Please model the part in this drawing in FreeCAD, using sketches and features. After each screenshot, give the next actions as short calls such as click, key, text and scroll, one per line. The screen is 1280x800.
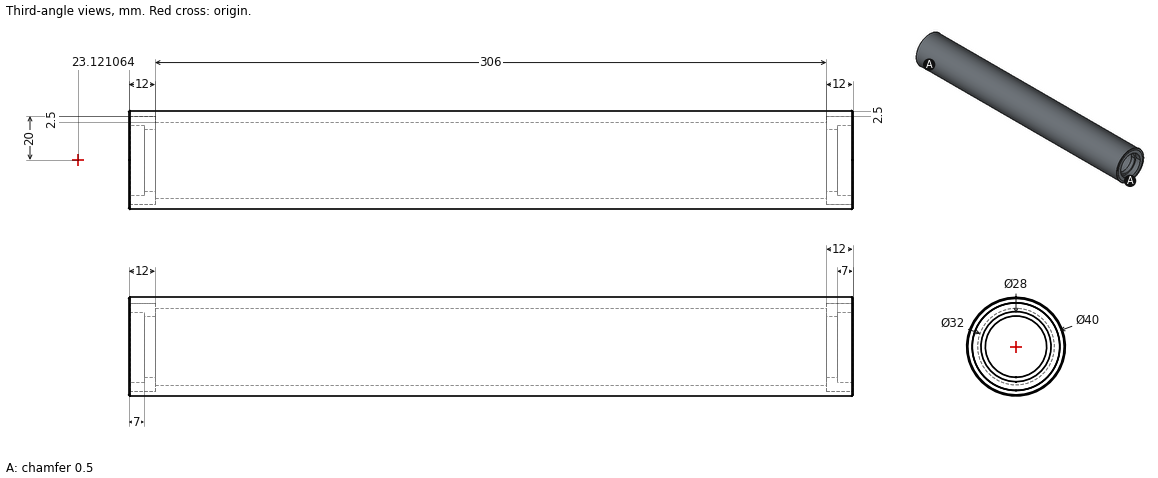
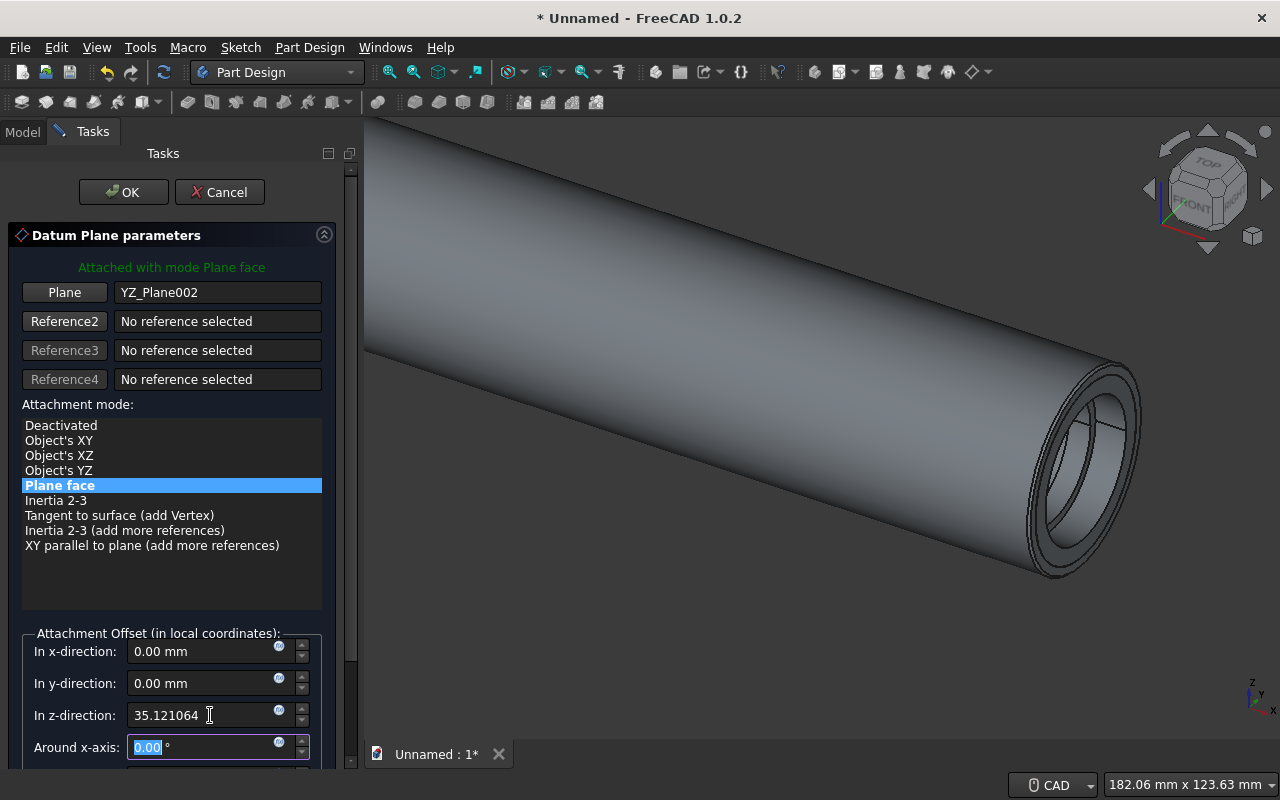
click(124, 192)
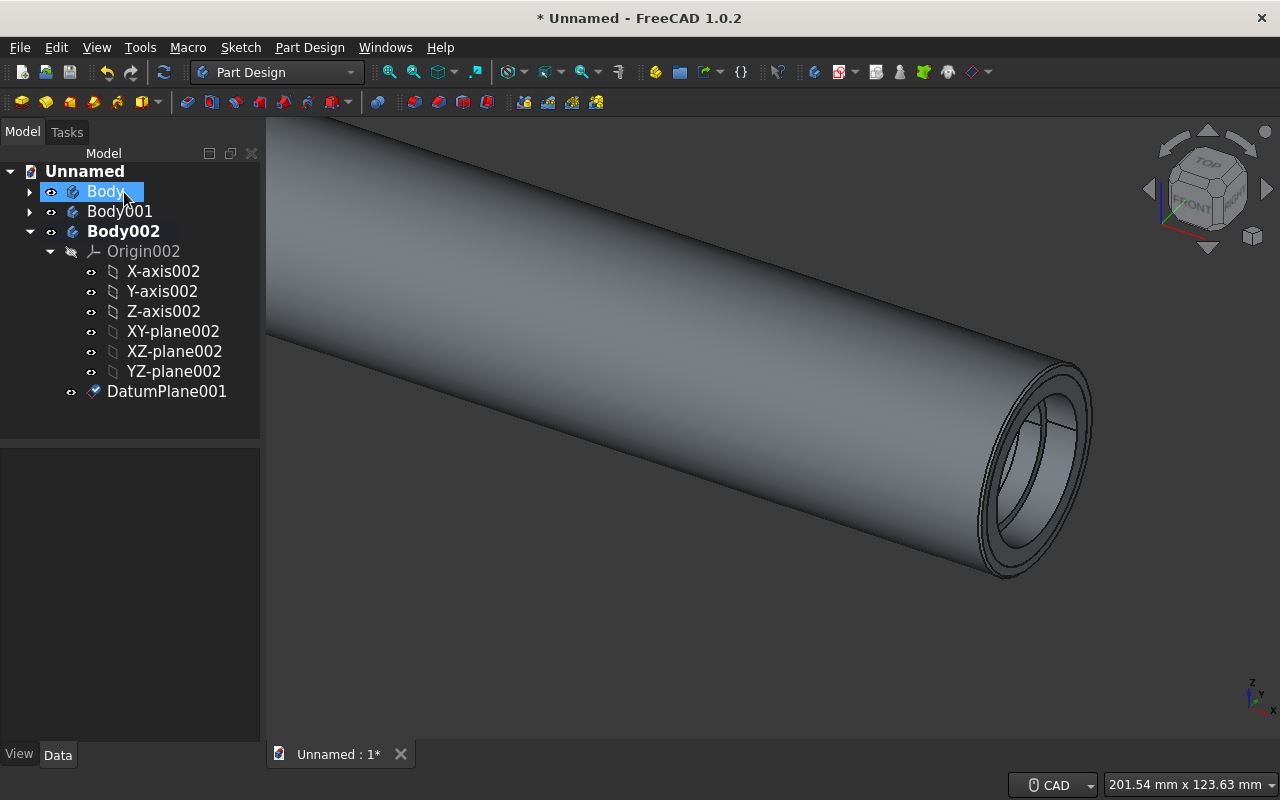
click(116, 392)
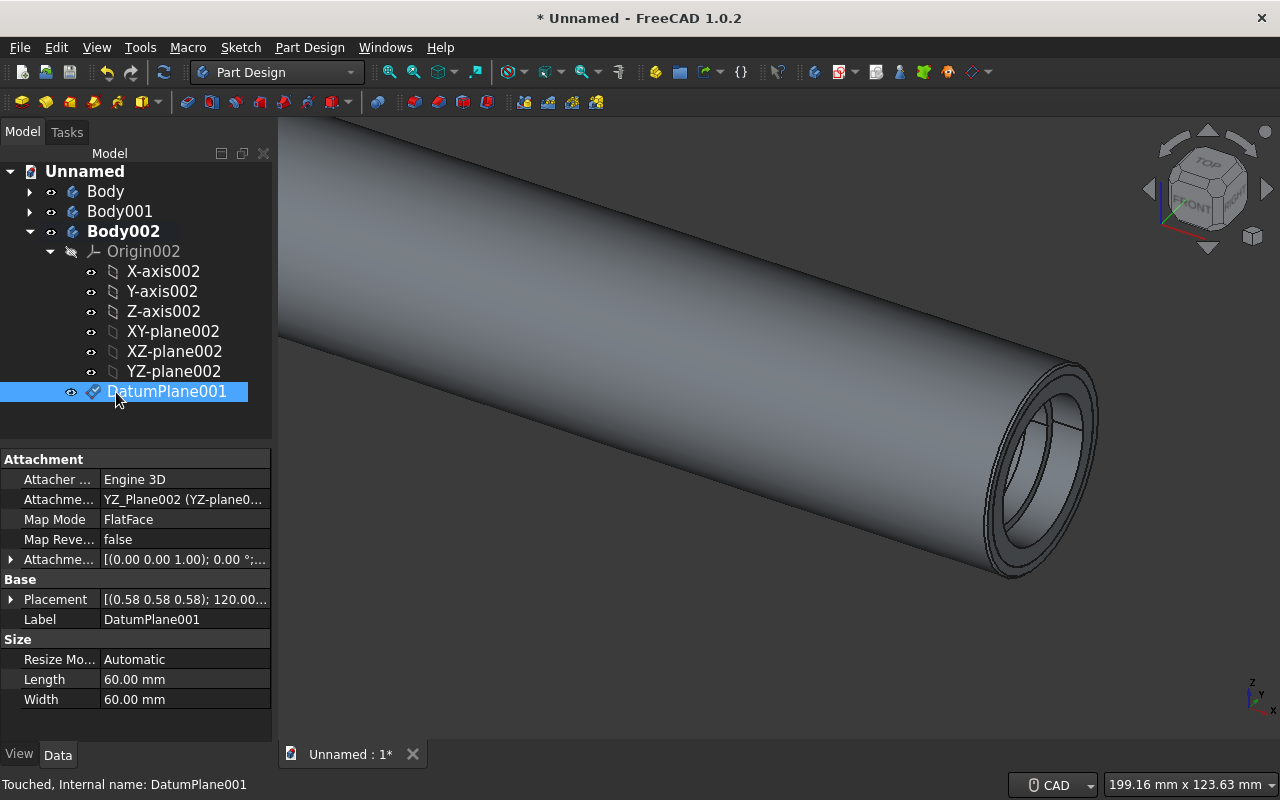
click(840, 72)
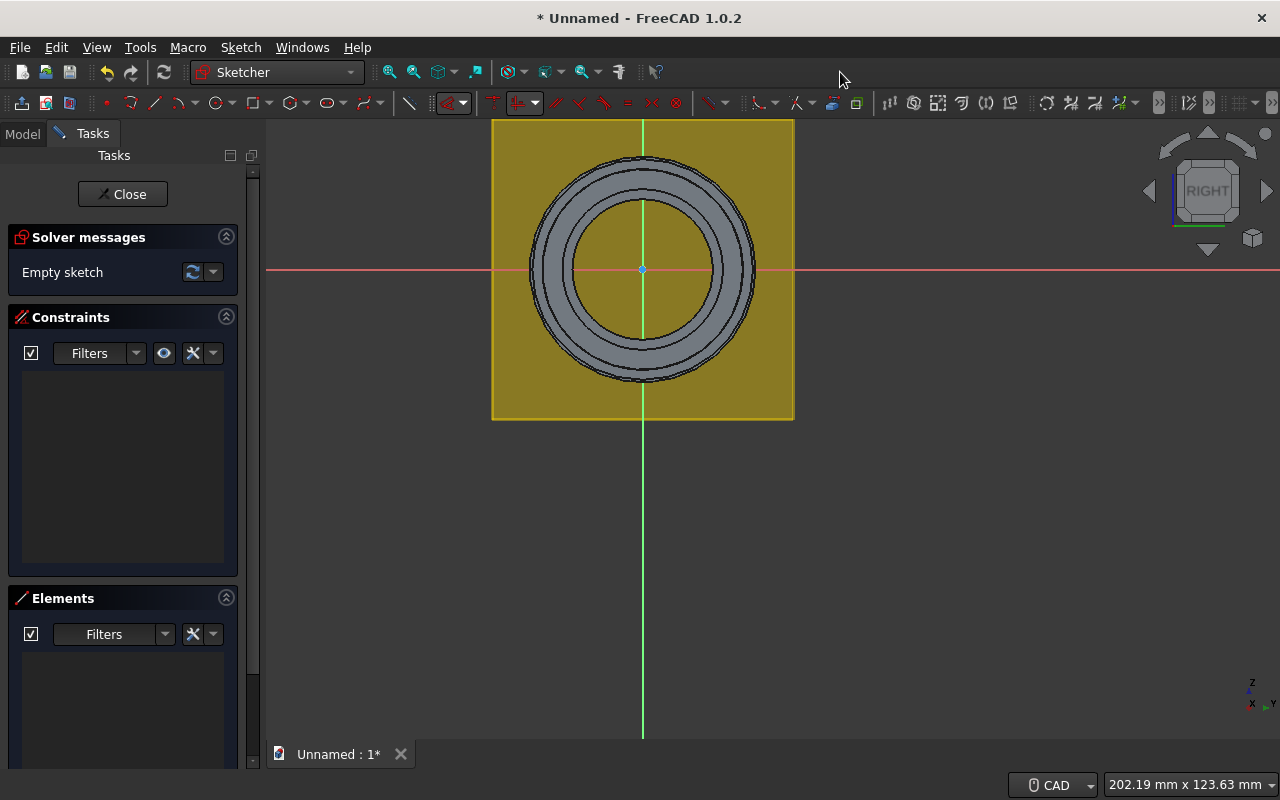
scroll(567, 147, up, 3)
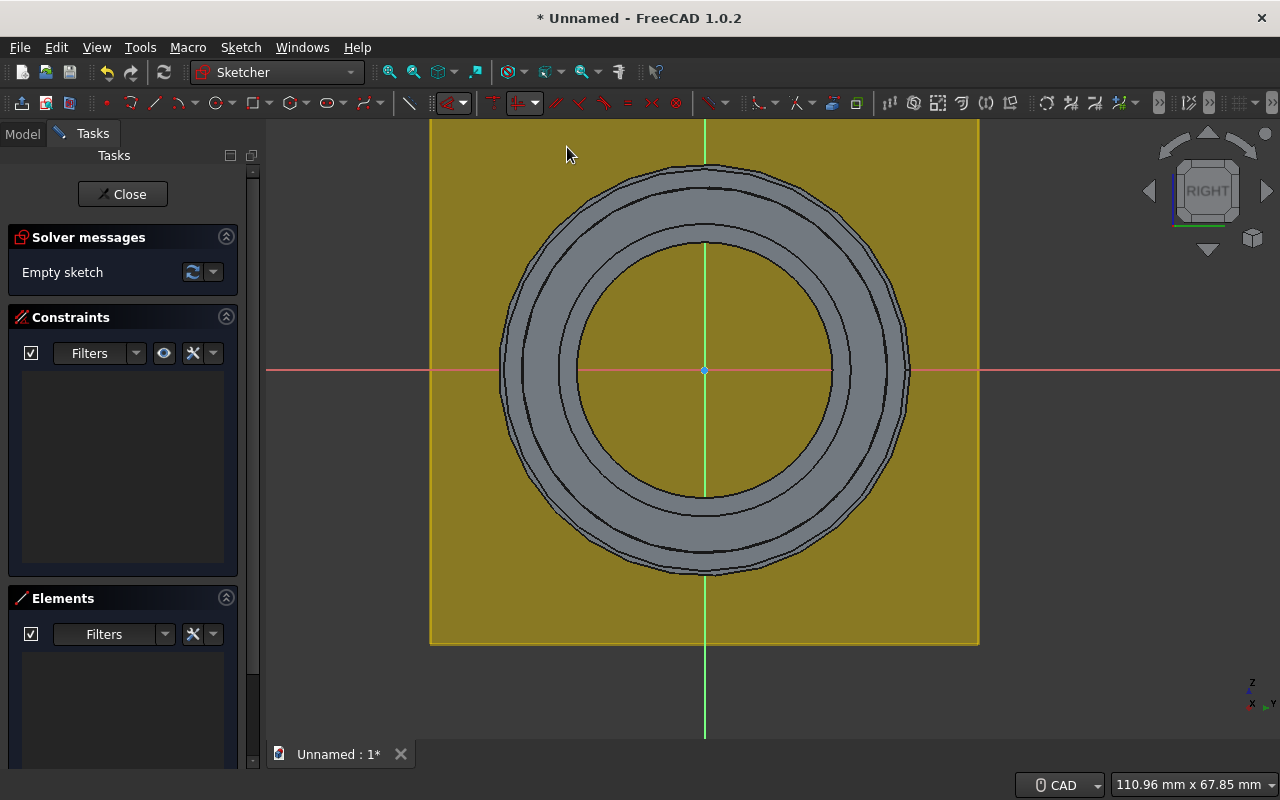
click(216, 104)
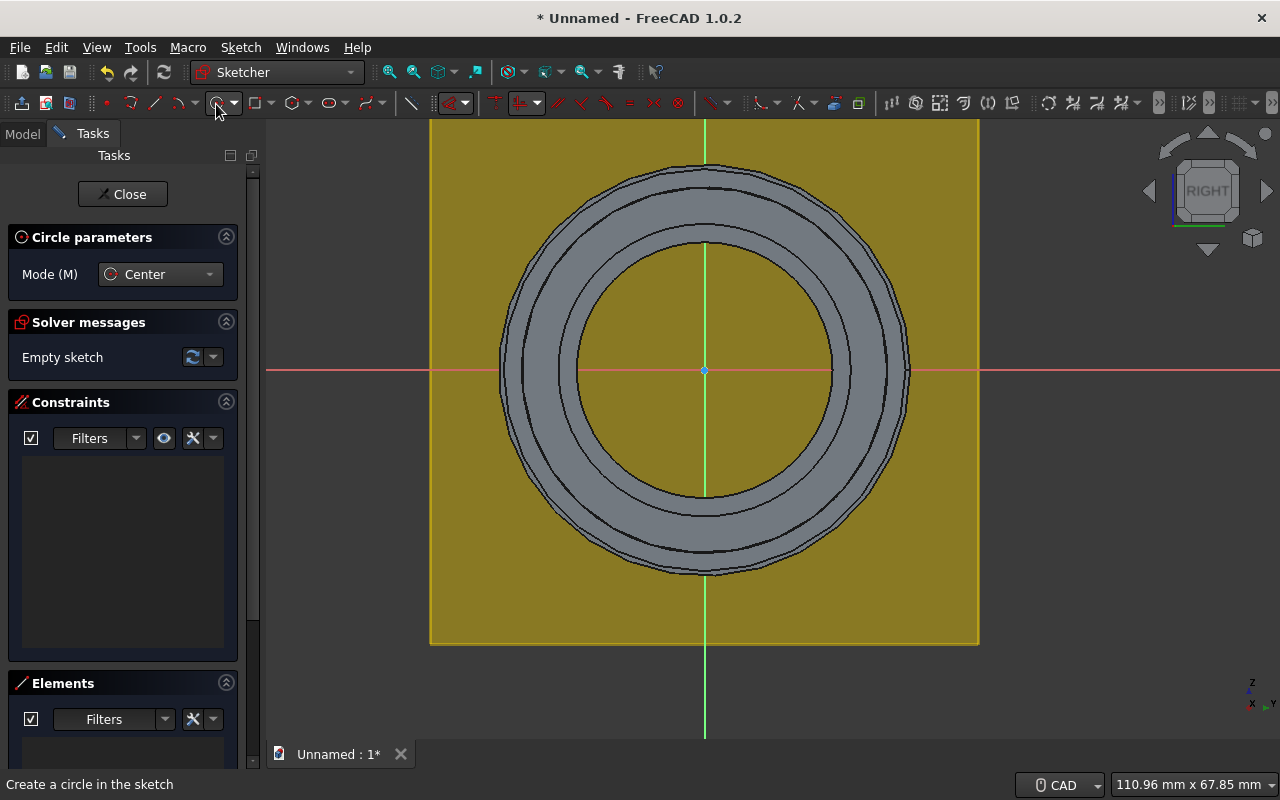
click(705, 370)
move(834, 241)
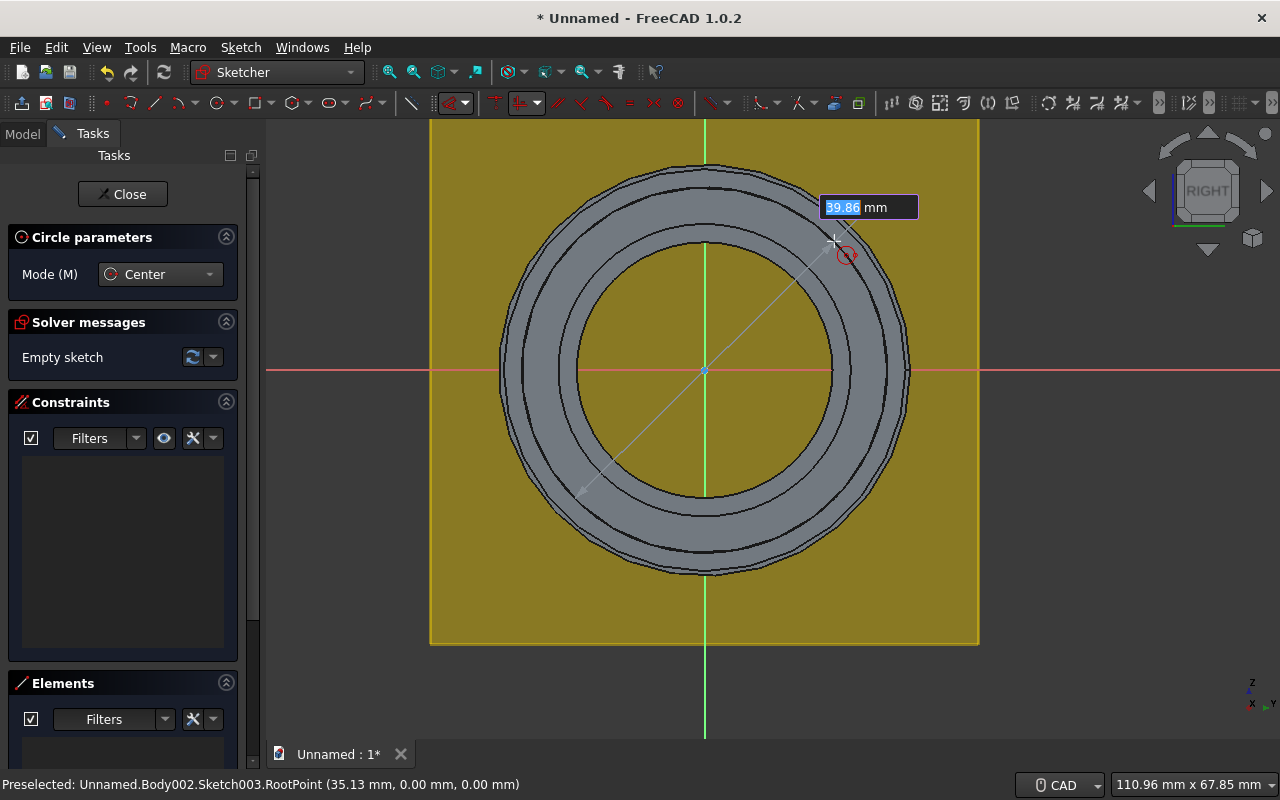
text(40)
key(Return)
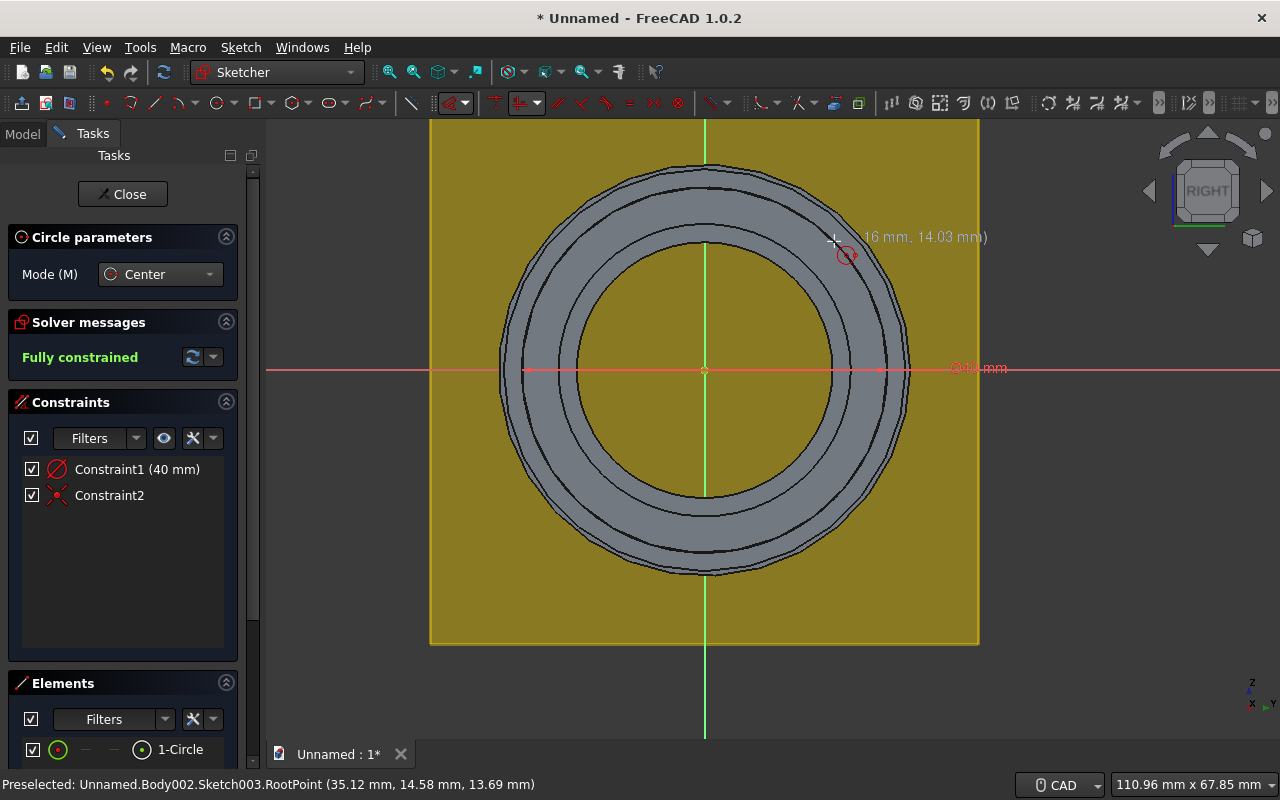
click(705, 370)
move(795, 280)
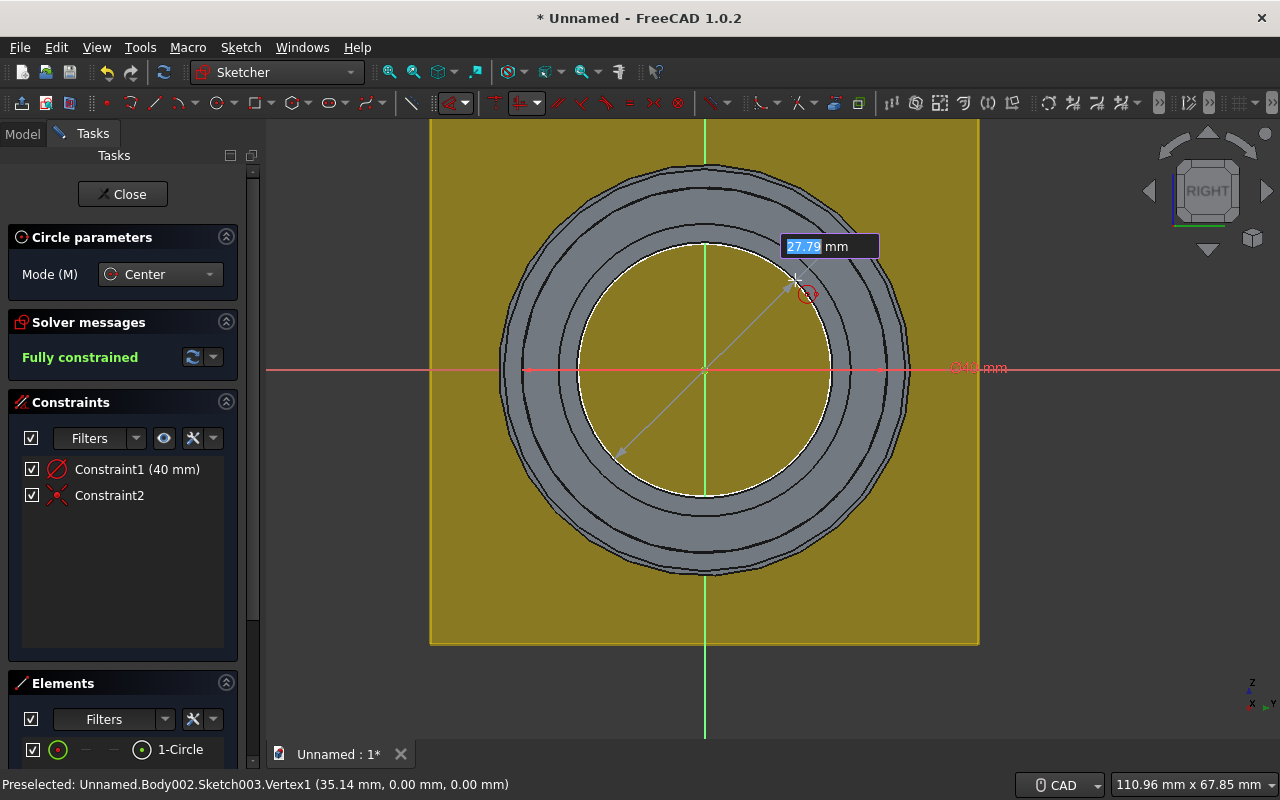
text(28)
key(Return)
key(Escape)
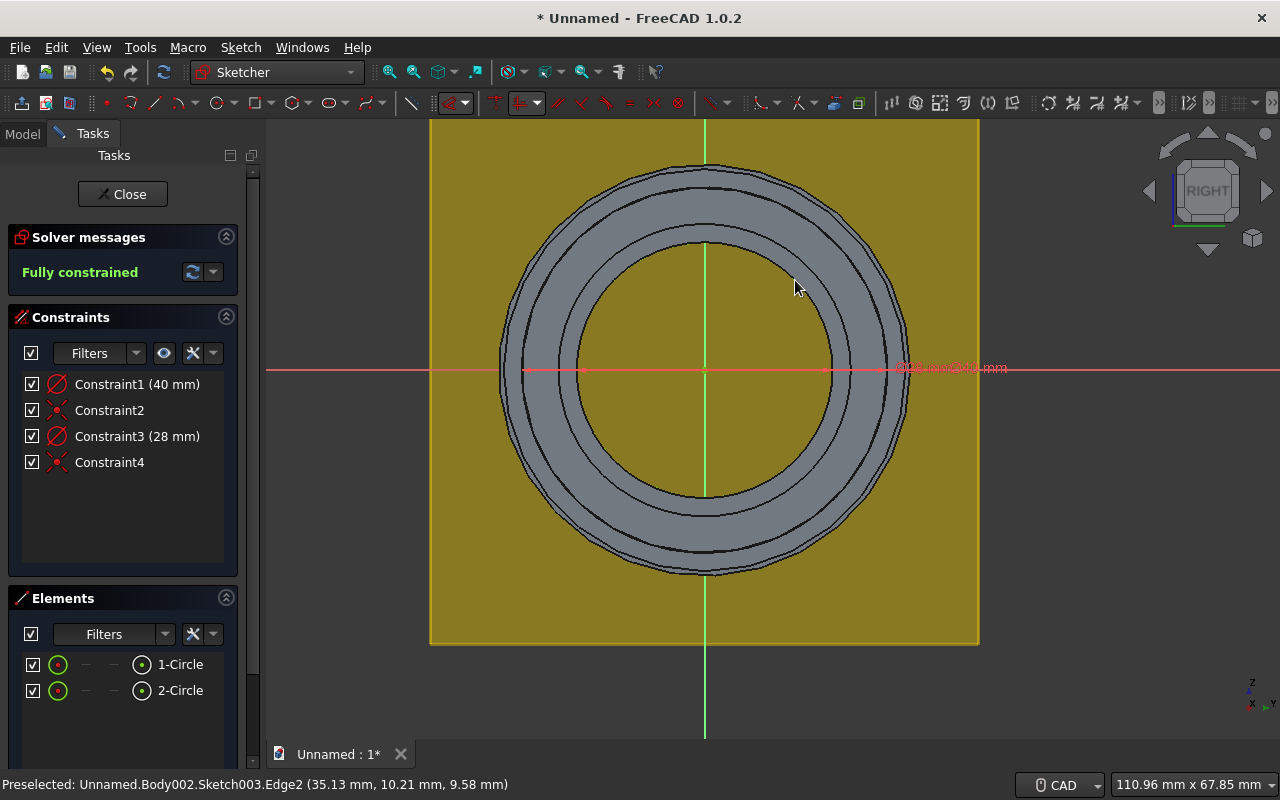
click(123, 194)